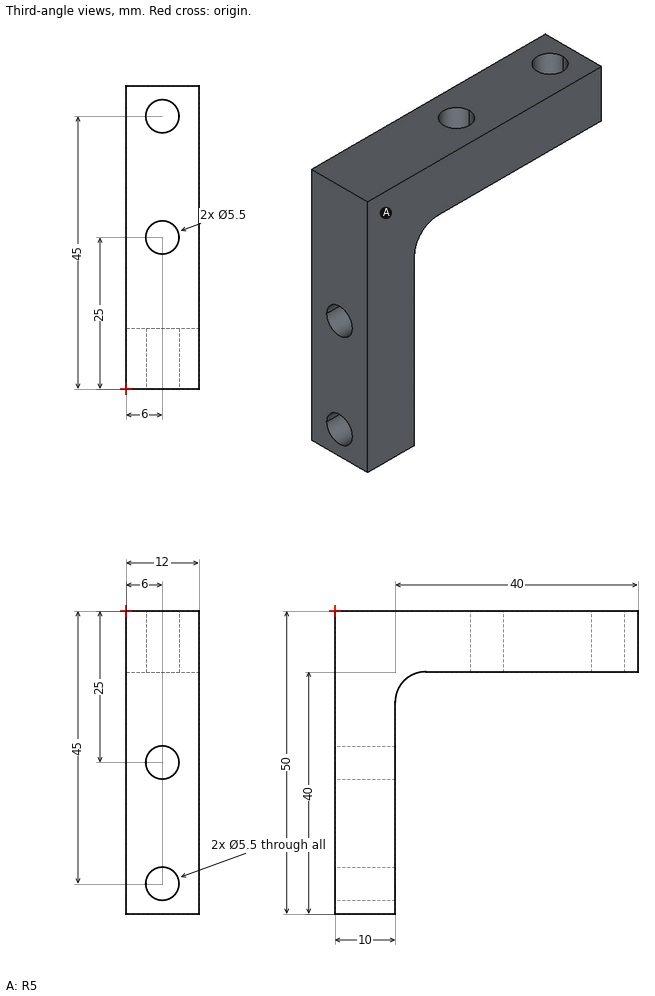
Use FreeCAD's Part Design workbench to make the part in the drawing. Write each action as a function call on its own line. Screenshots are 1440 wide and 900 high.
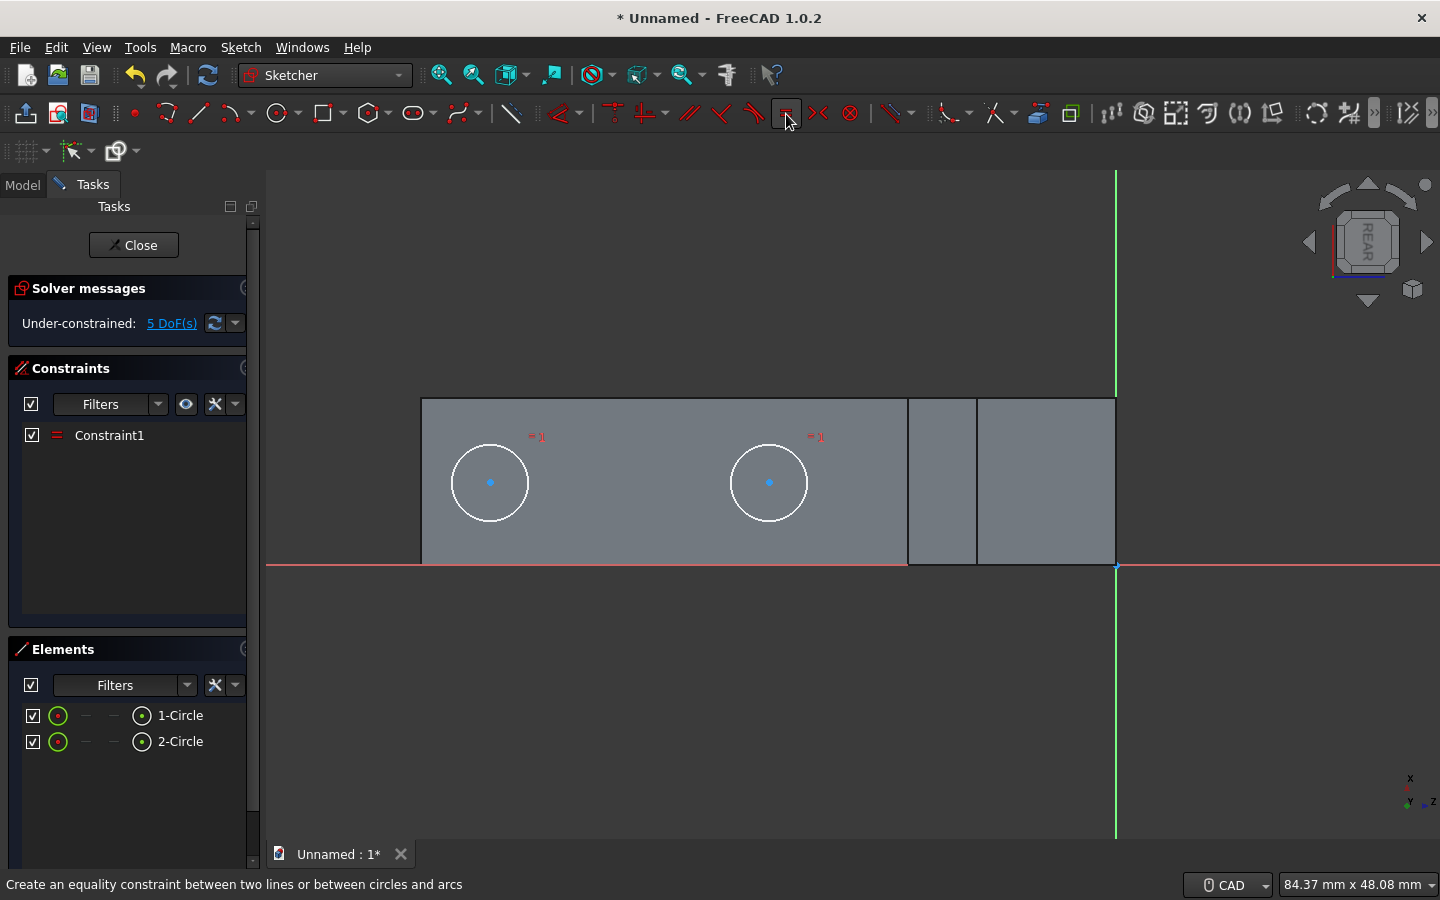
click(558, 114)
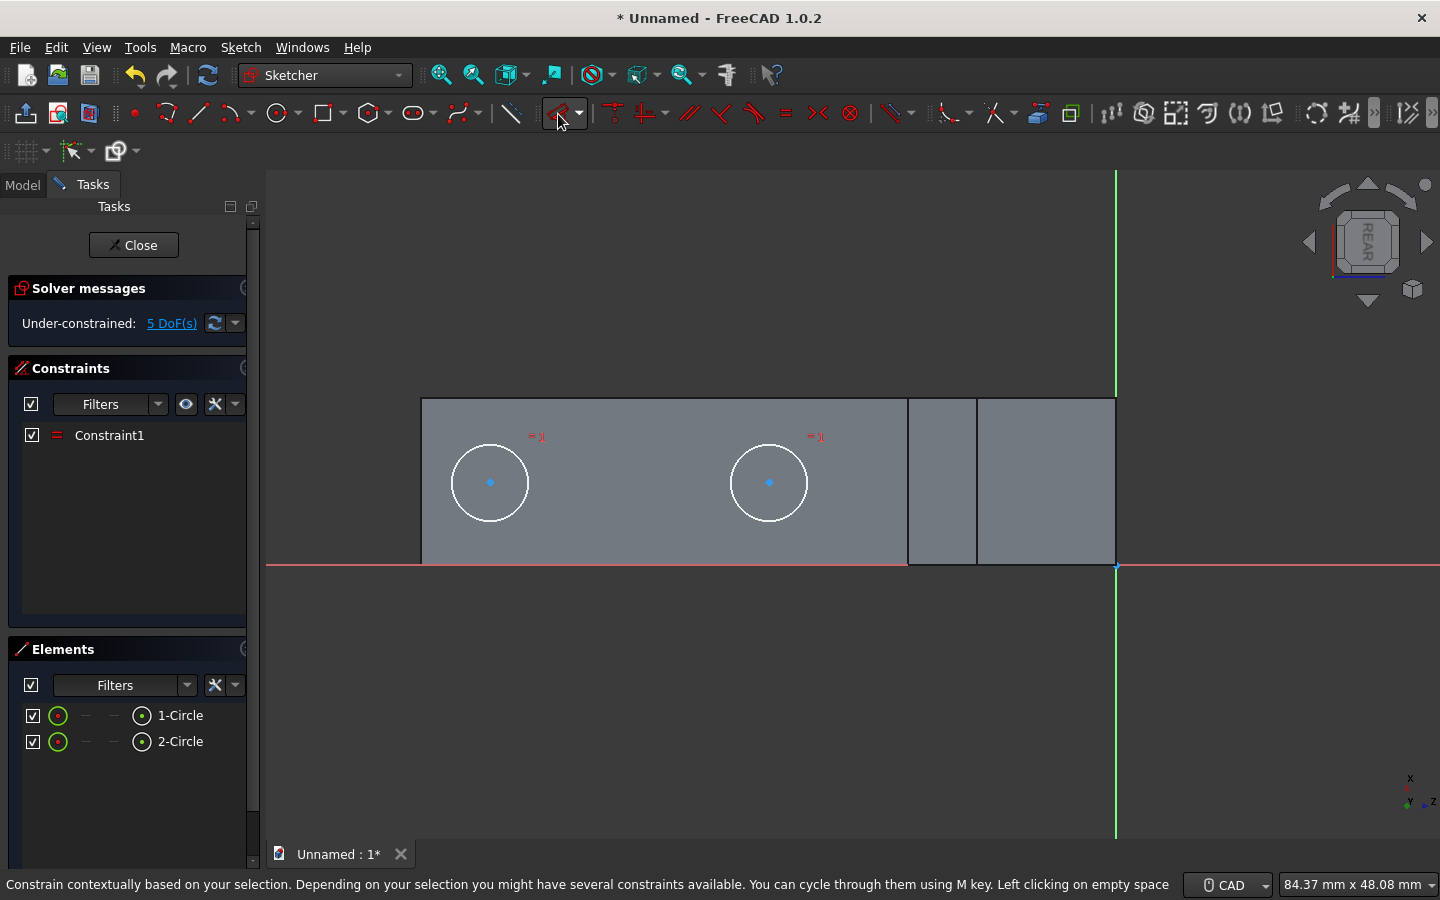
click(517, 456)
click(540, 433)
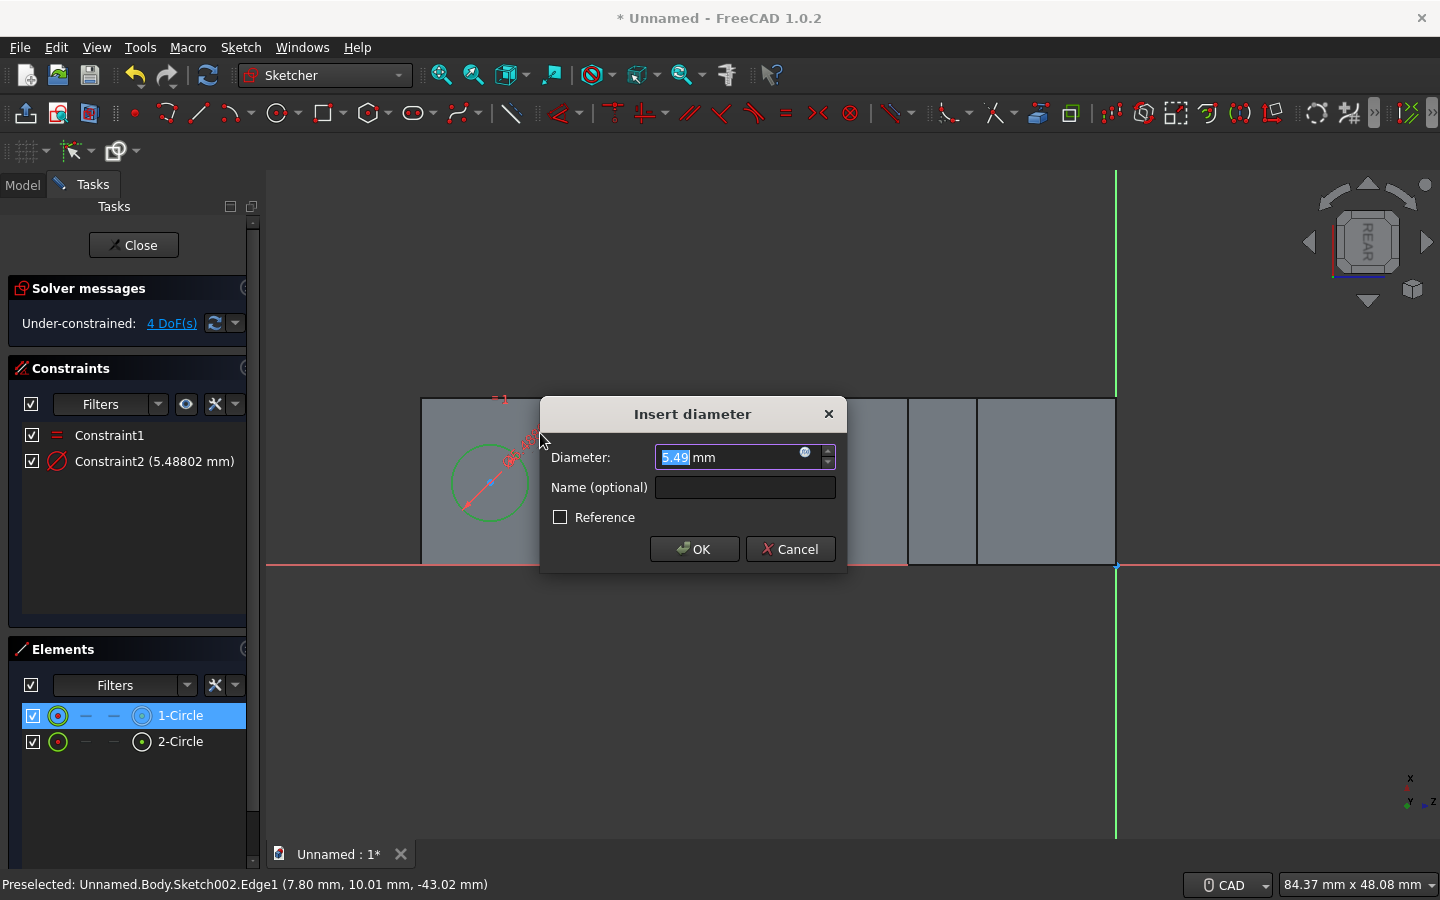
text(5.5)
key(Return)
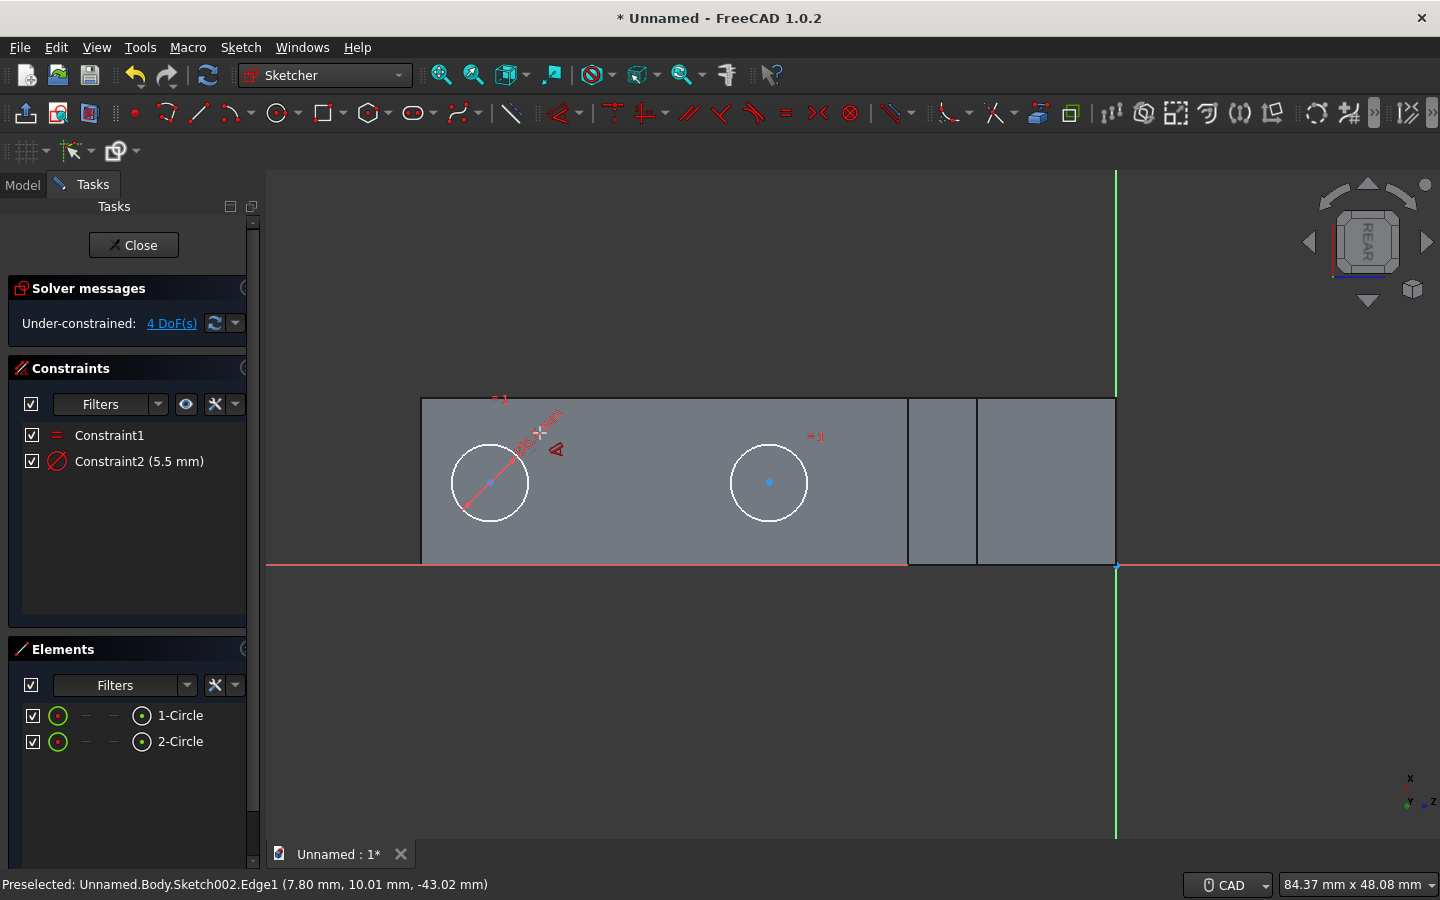
click(490, 483)
click(1150, 524)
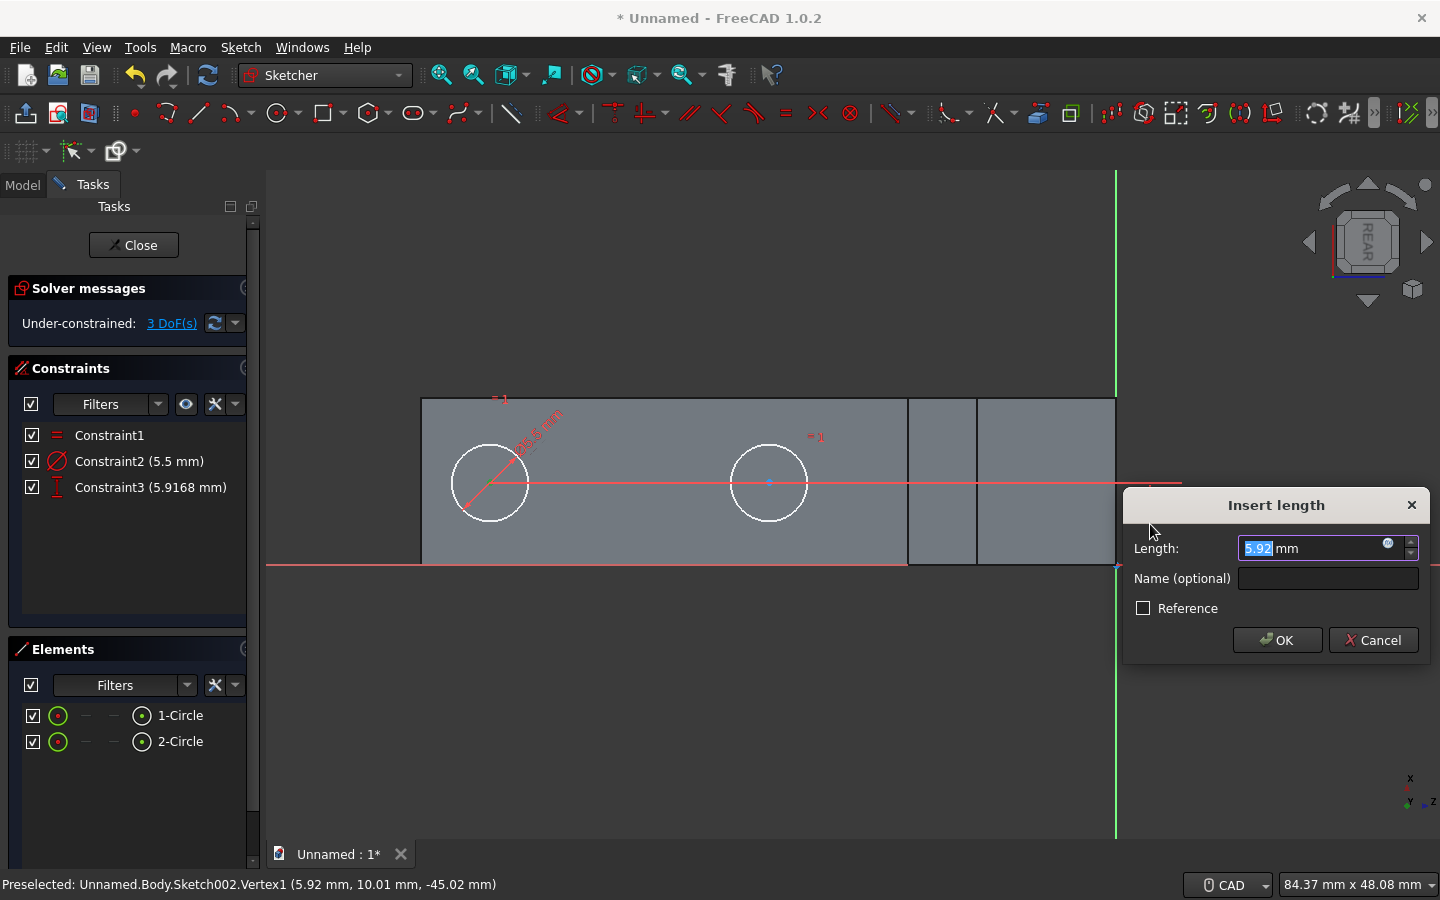
text(6)
key(Return)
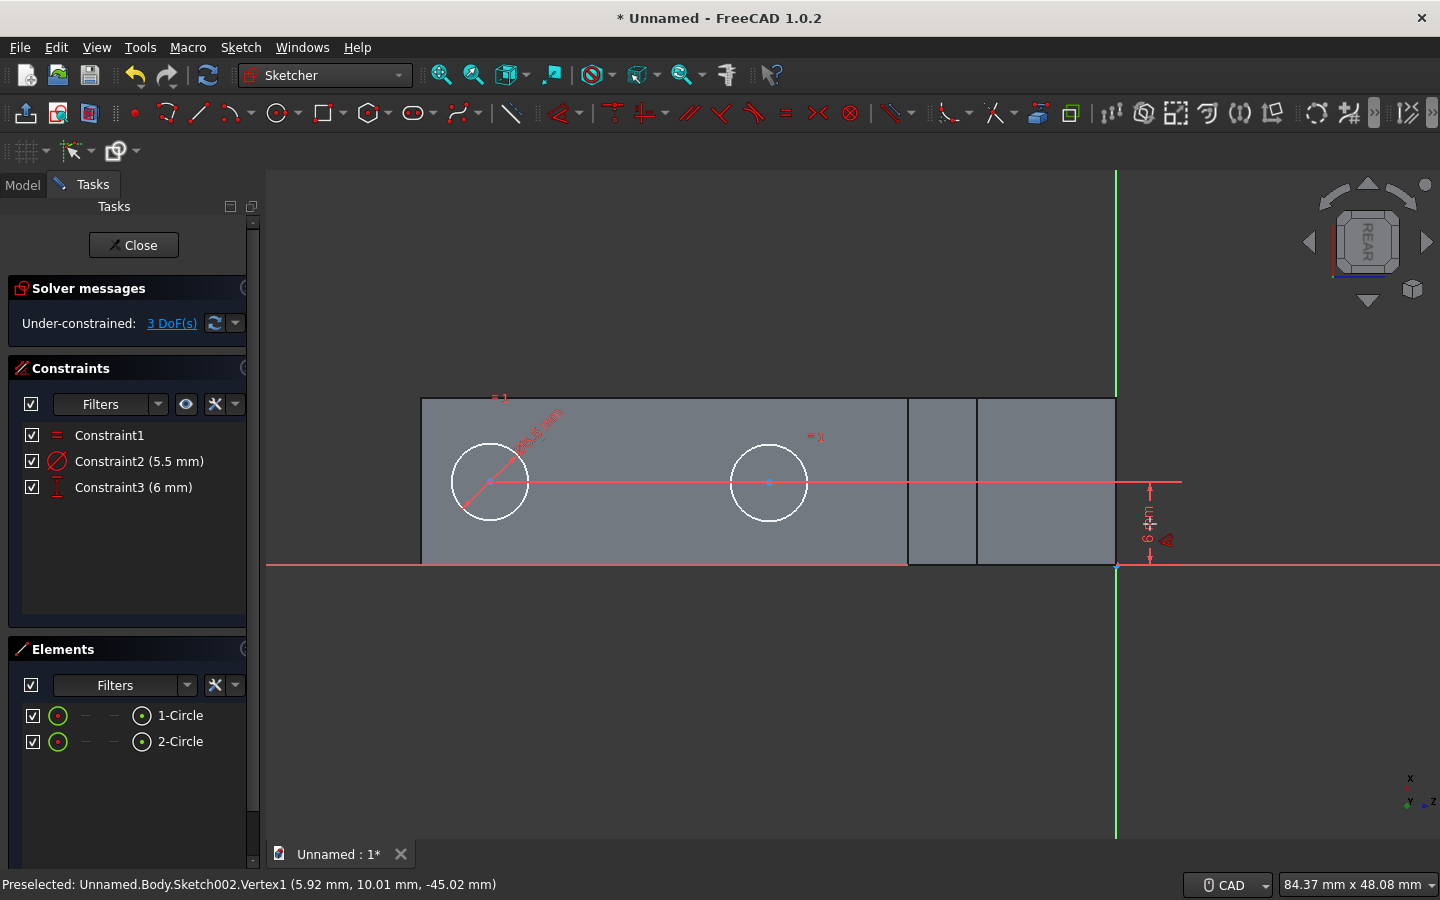
click(769, 483)
click(1150, 495)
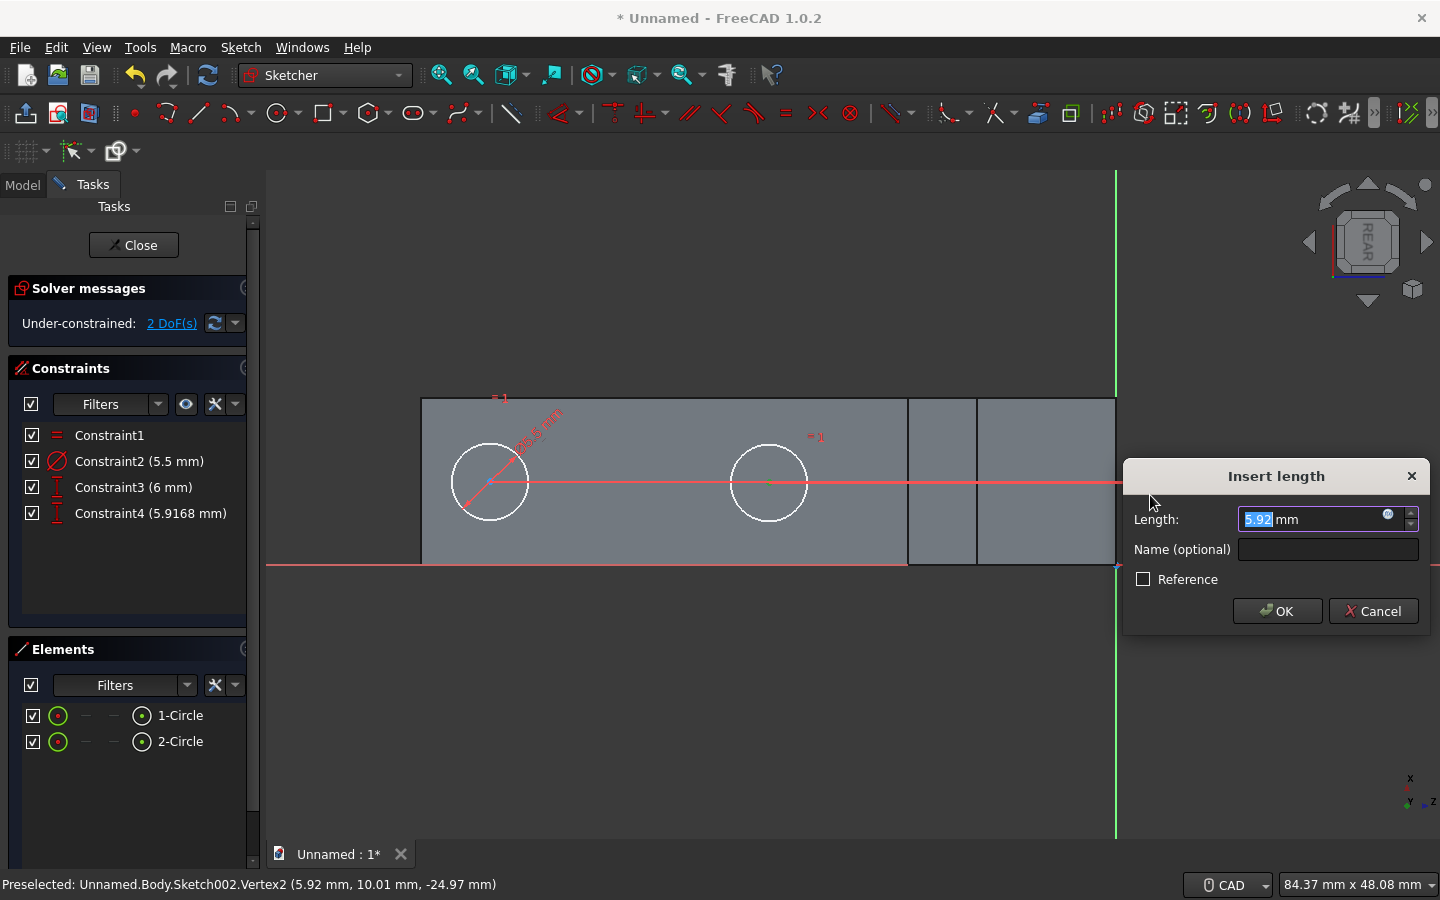
text(6)
key(Return)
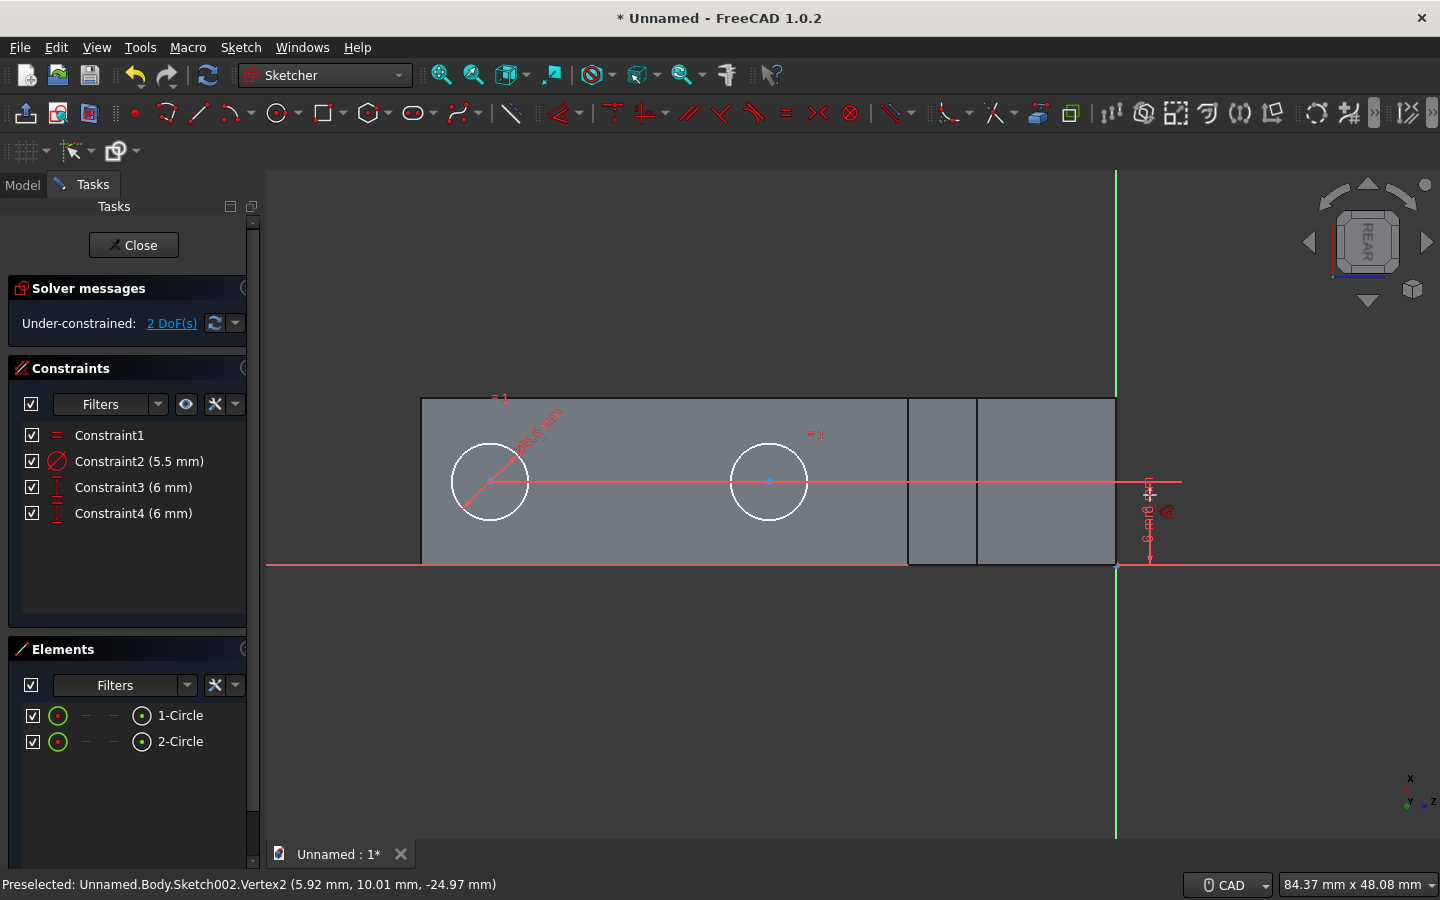
click(490, 482)
click(803, 599)